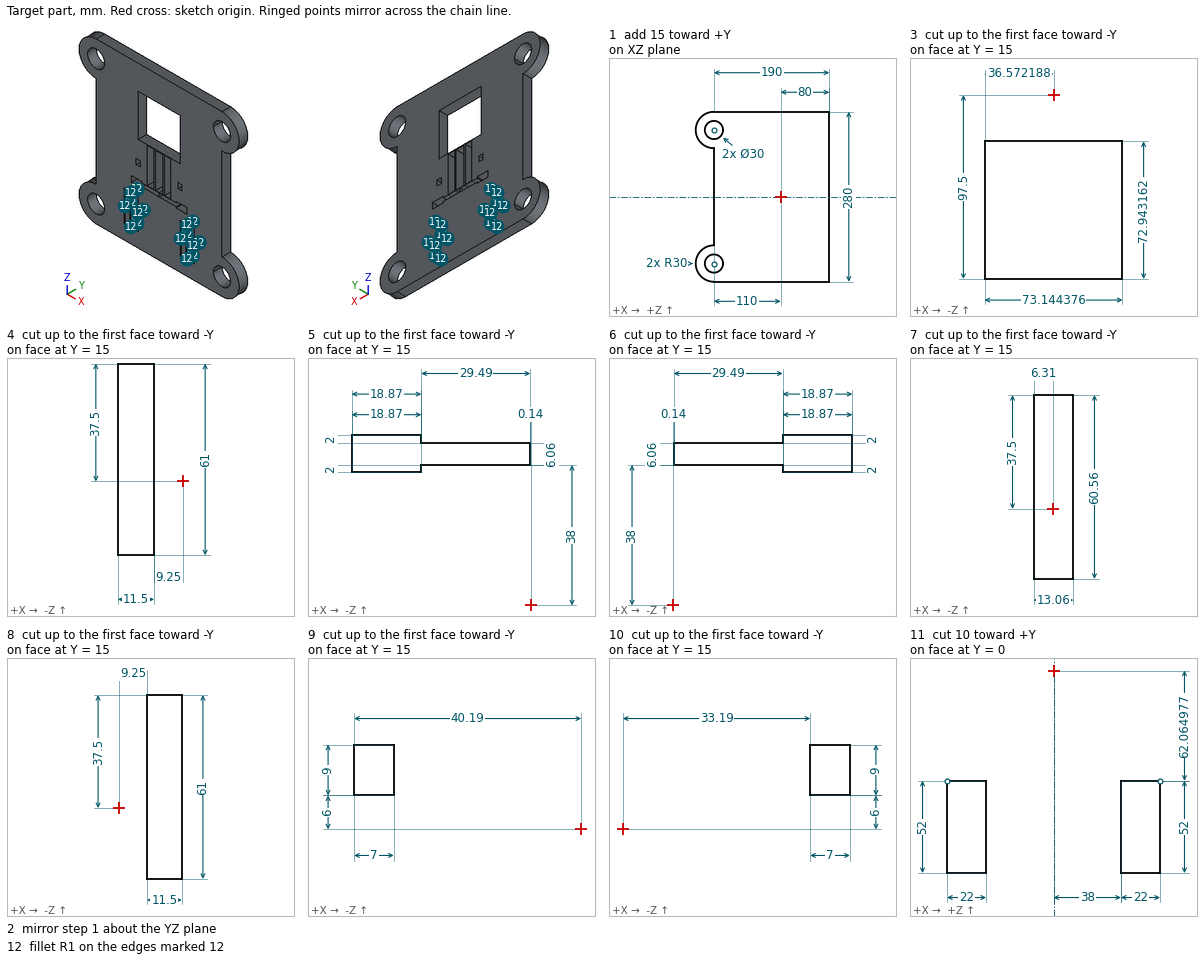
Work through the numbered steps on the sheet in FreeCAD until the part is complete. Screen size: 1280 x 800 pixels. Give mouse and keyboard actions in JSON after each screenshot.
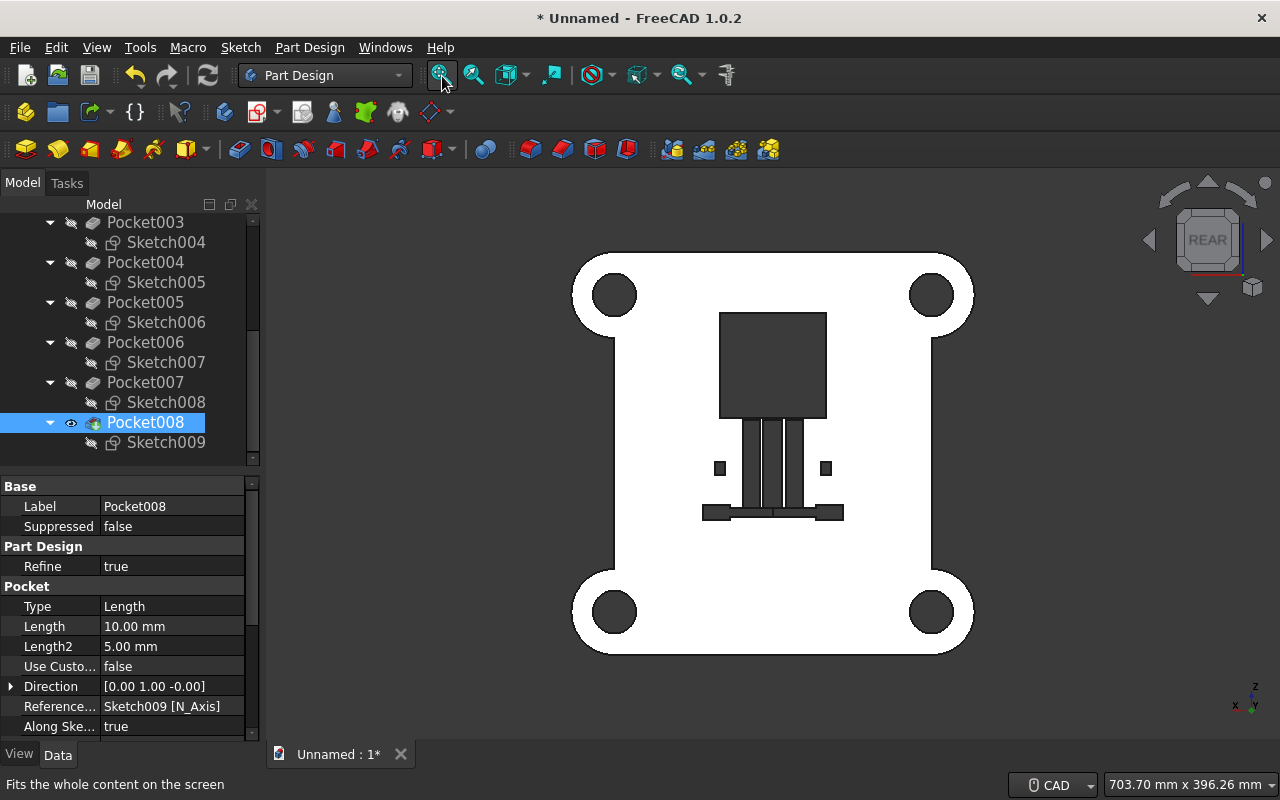
{"action": "key", "text": "6"}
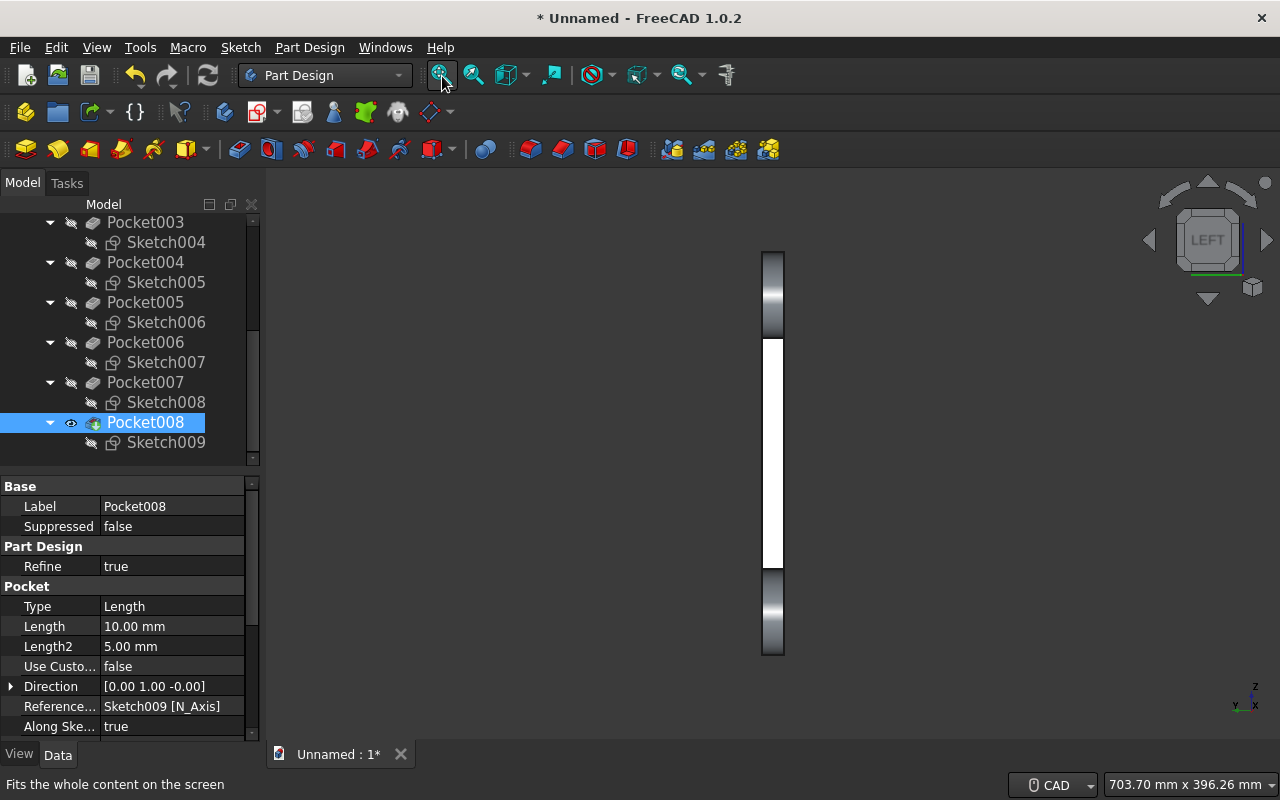
{"action": "key", "text": "v 3"}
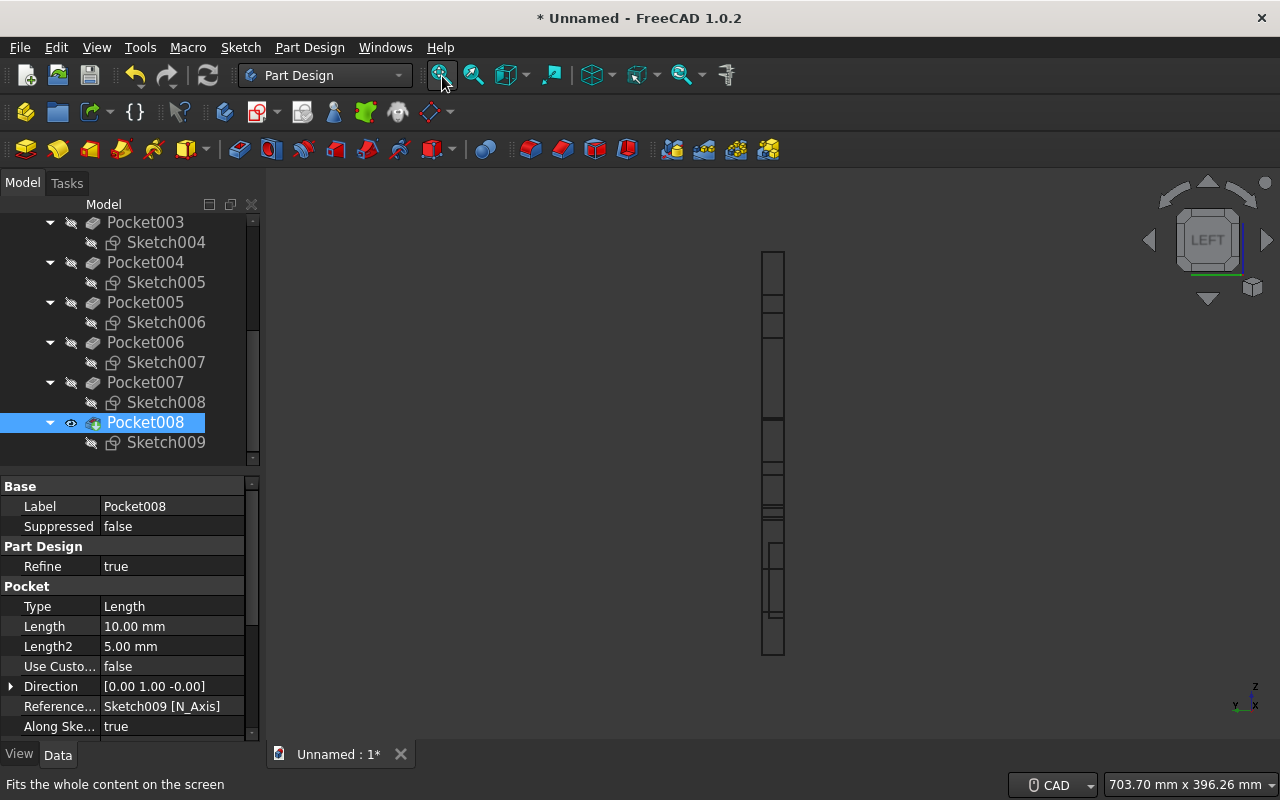
{"action": "key", "text": "0"}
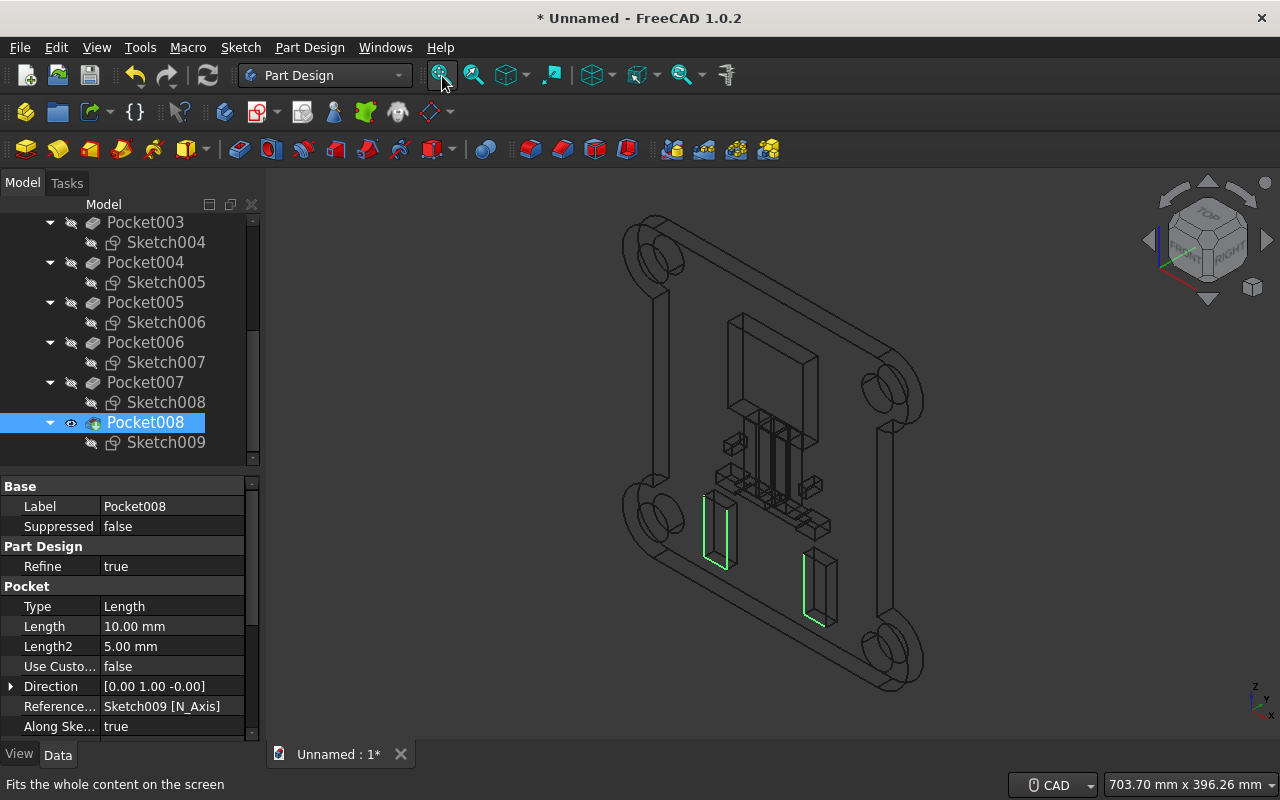
{"action": "left_click", "coordinate": [826, 596], "text": "ctrl"}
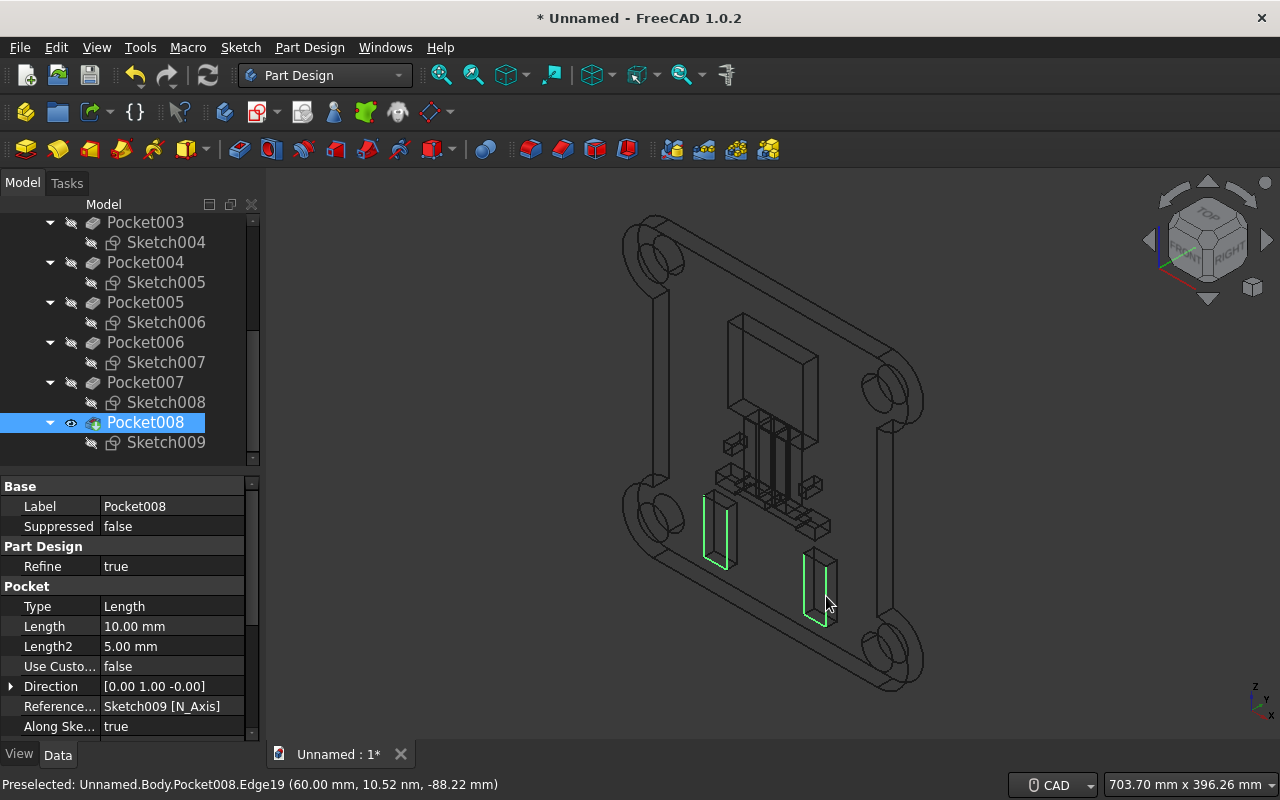
{"action": "left_click", "coordinate": [815, 559], "text": "ctrl"}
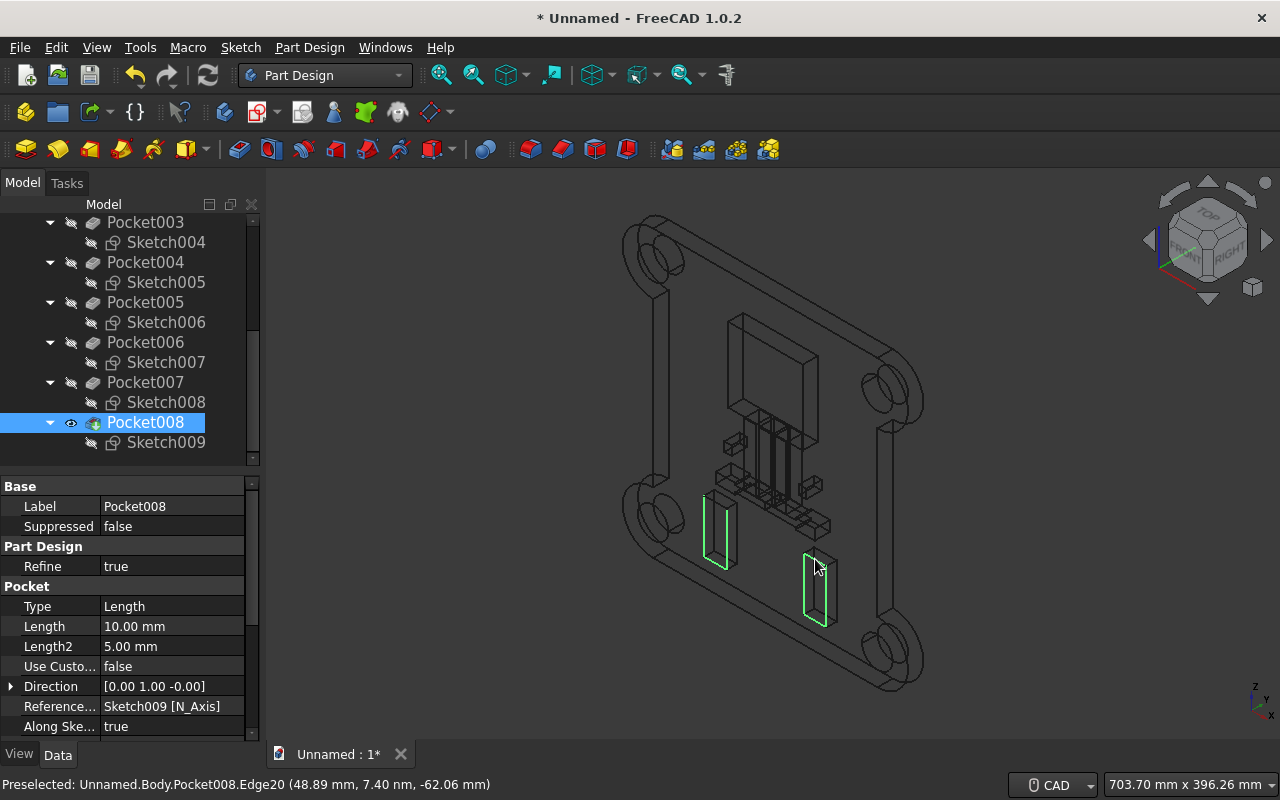
{"action": "left_click", "coordinate": [715, 501], "text": "ctrl"}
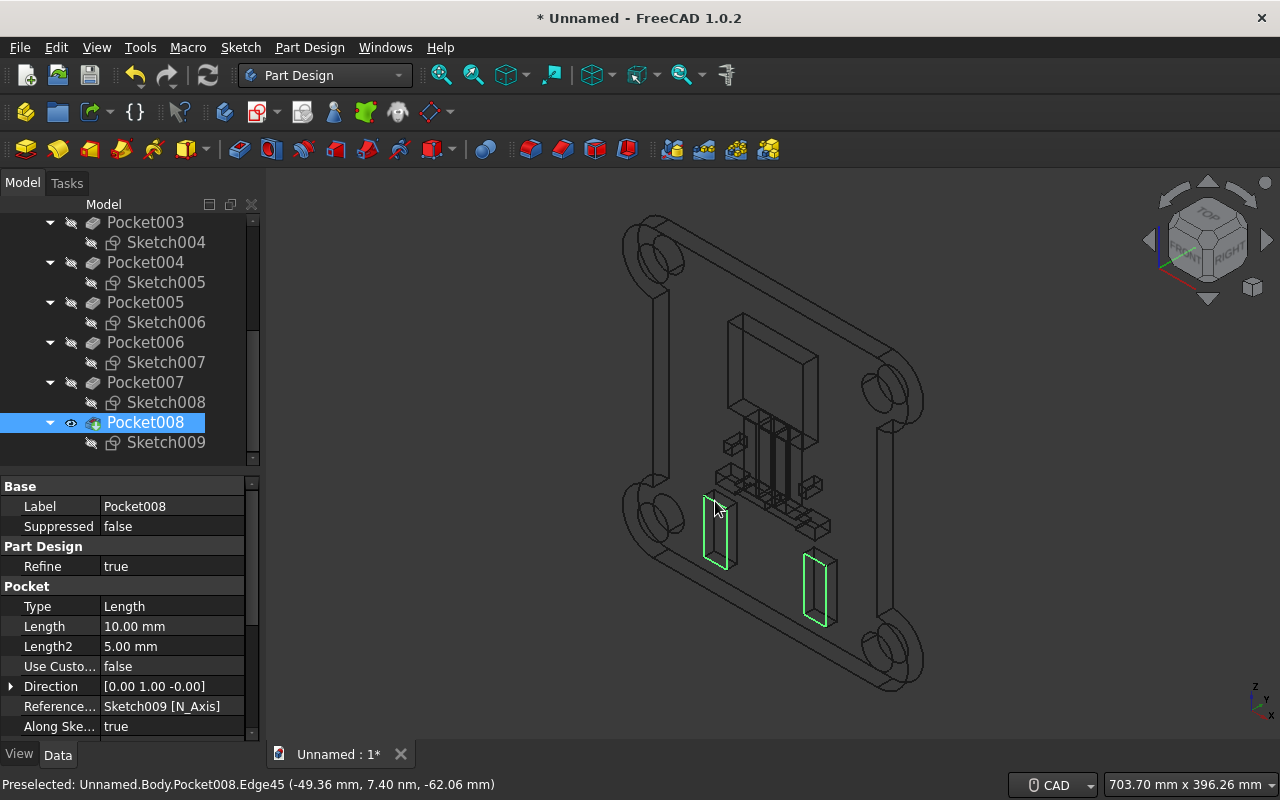
{"action": "key", "text": "v 1"}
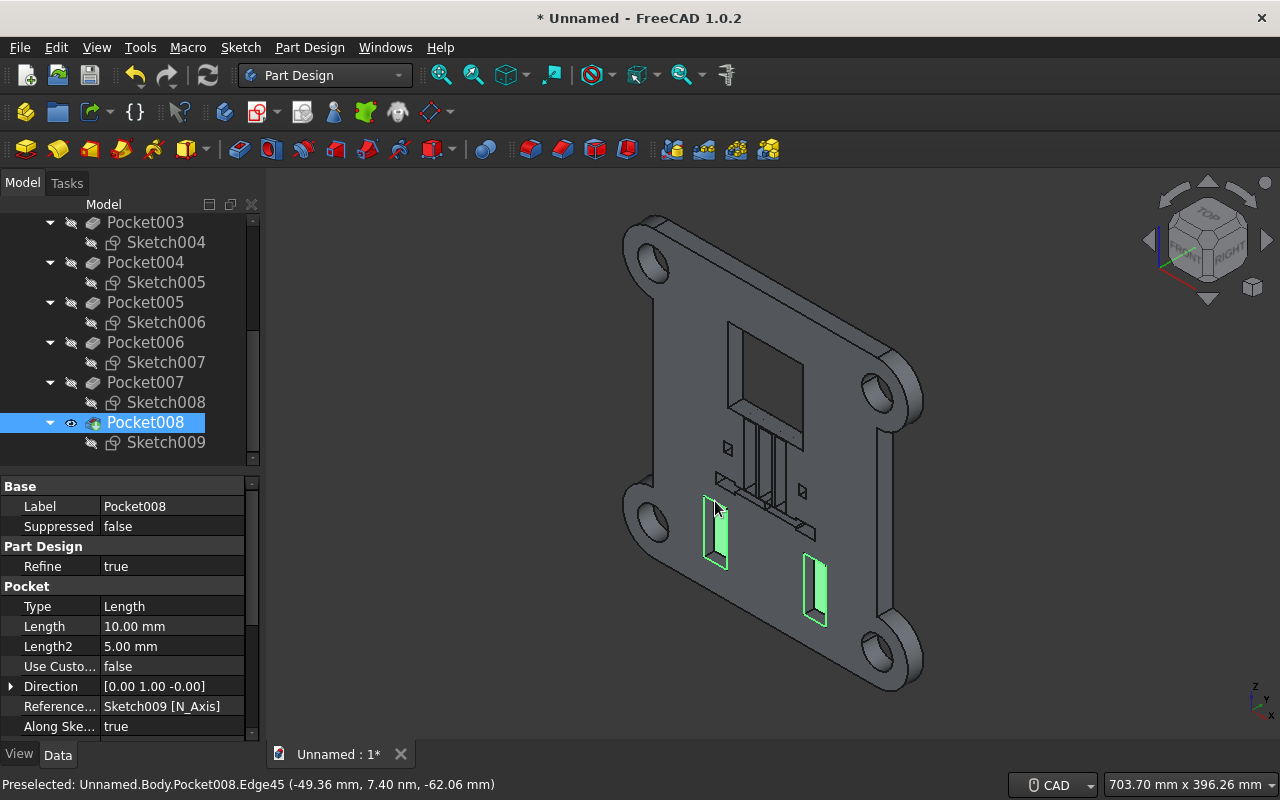
{"action": "left_click", "coordinate": [532, 150]}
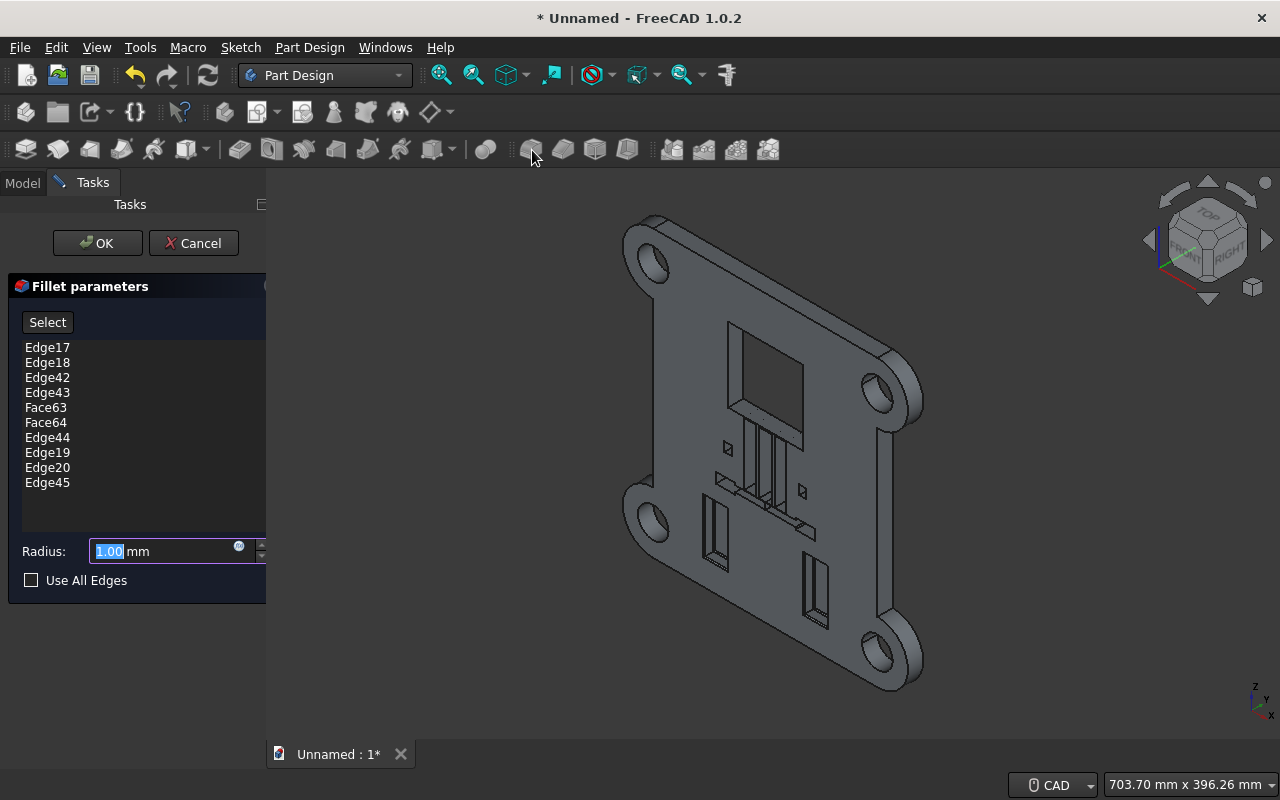
{"action": "type", "text": "1"}
{"action": "key", "text": "Tab"}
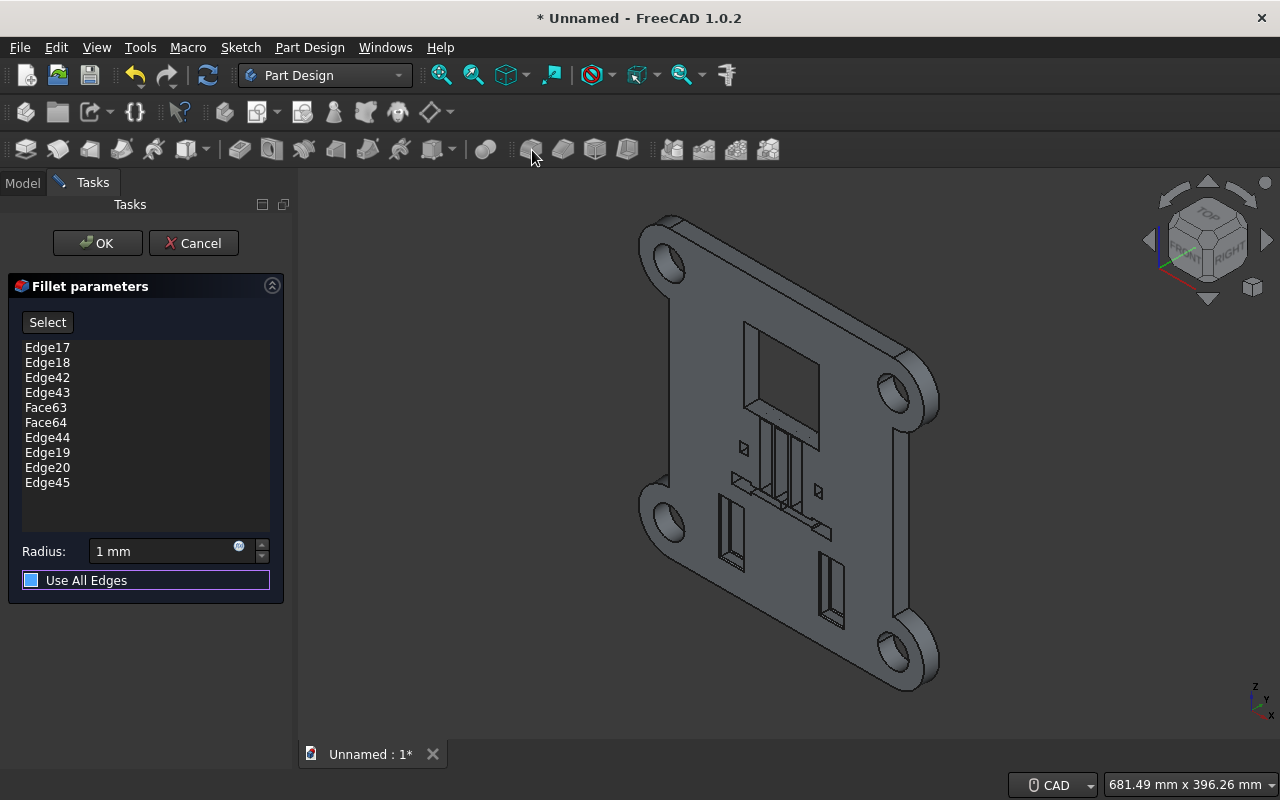
{"action": "left_click", "coordinate": [98, 243]}